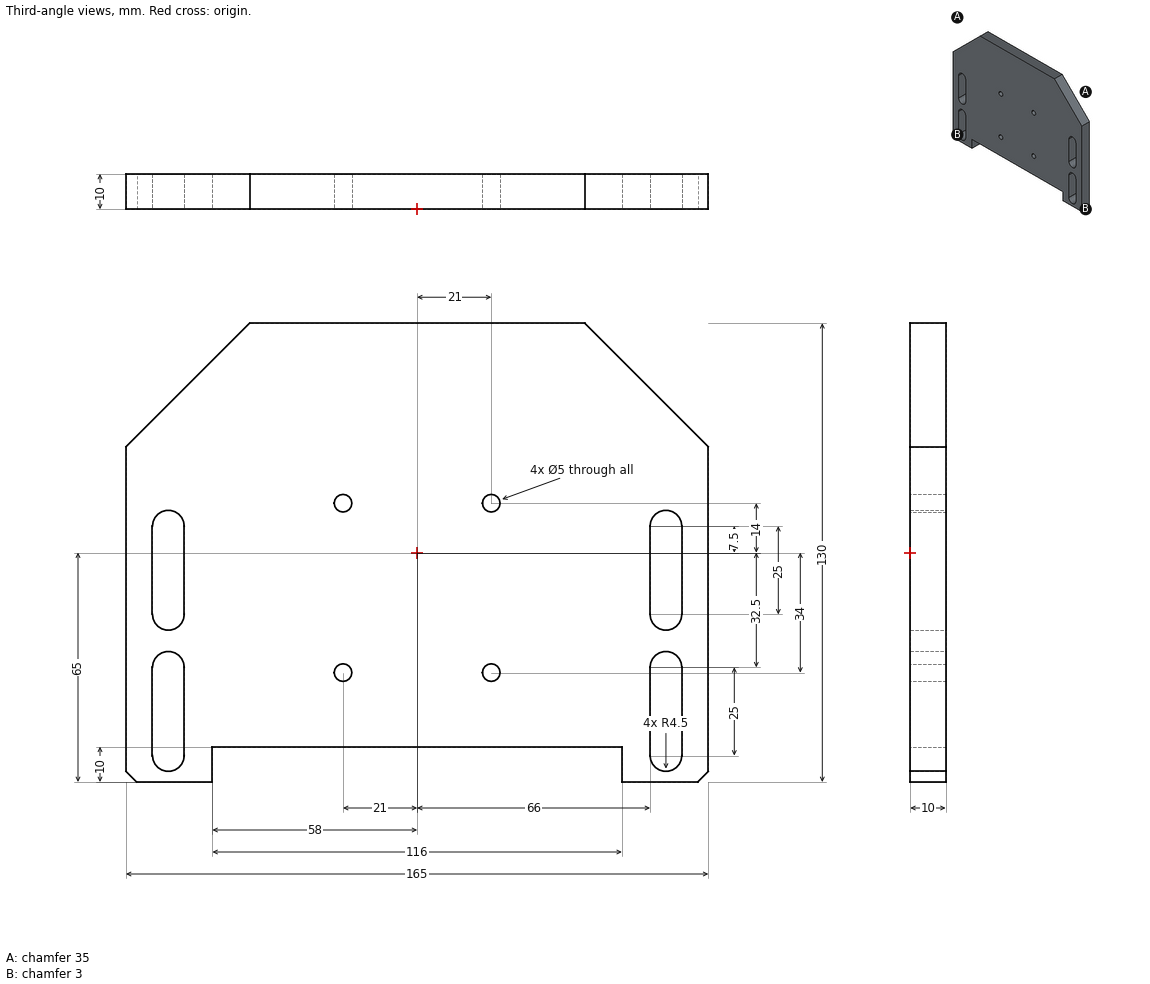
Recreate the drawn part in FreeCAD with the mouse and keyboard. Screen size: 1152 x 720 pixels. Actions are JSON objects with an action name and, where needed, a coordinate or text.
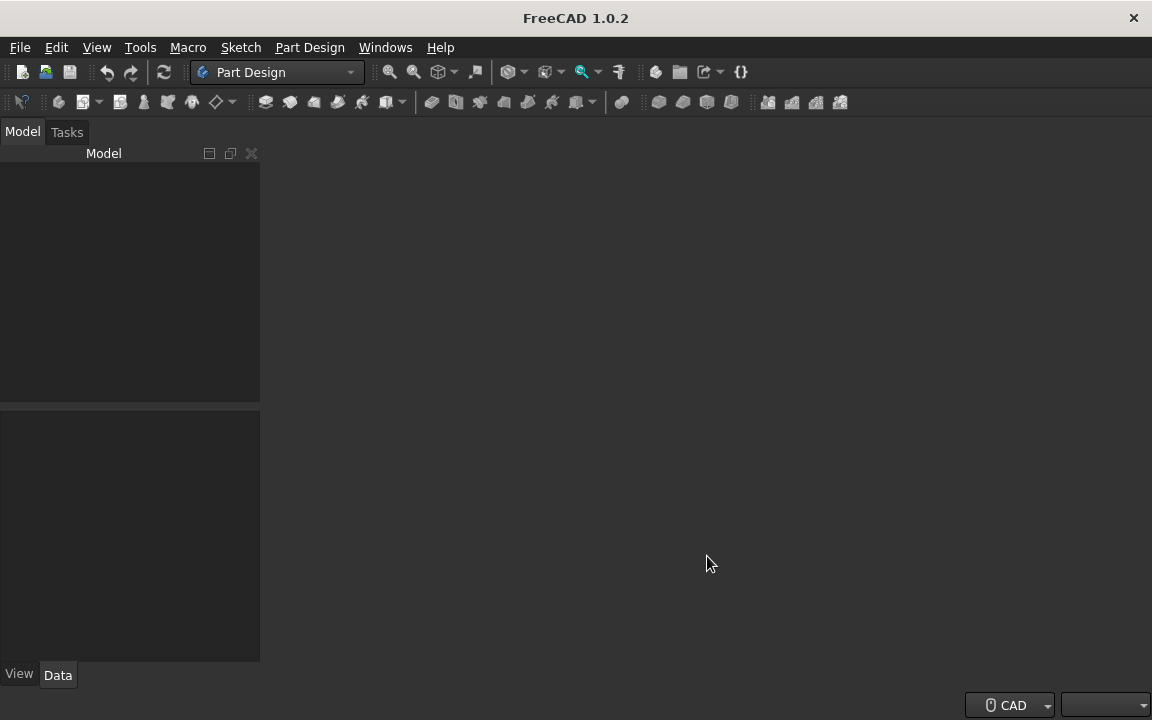
{"action": "key", "text": "ctrl+n"}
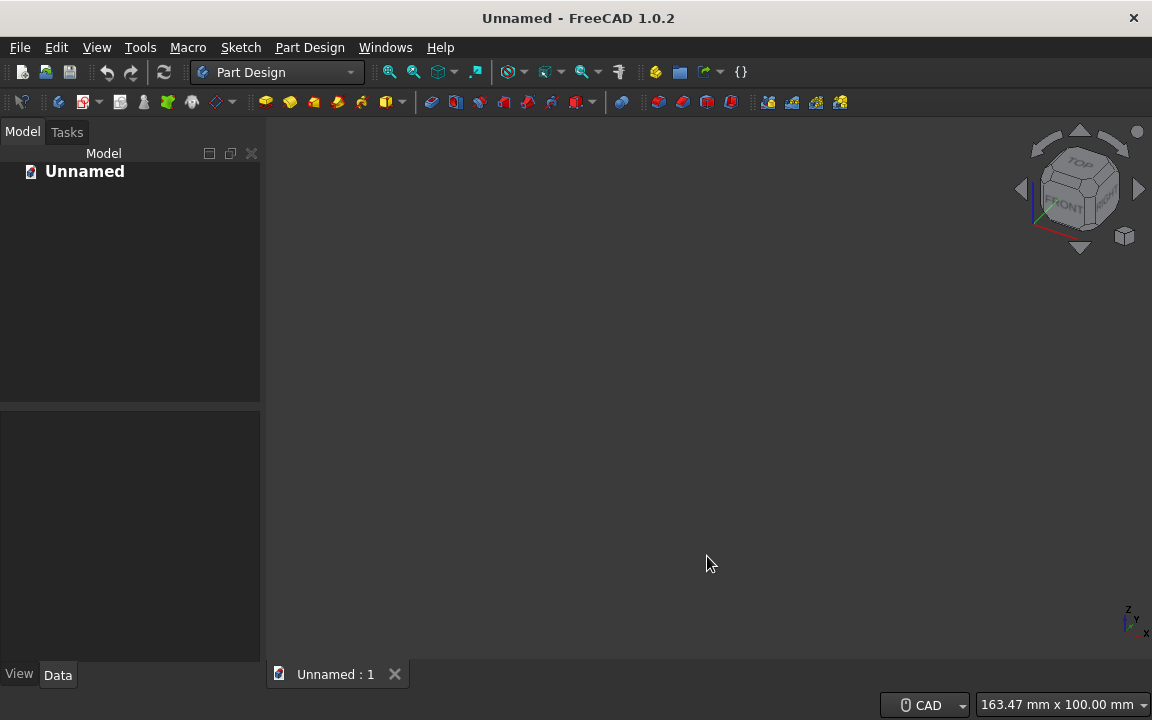
{"action": "left_click", "coordinate": [84, 102]}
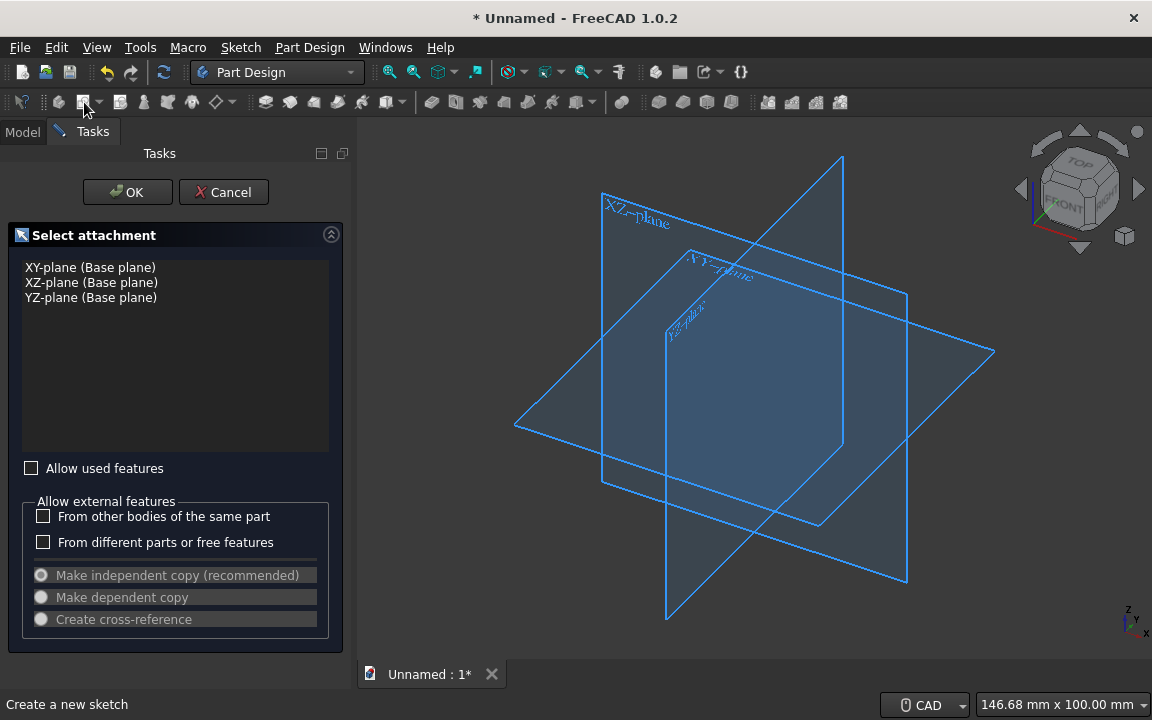
{"action": "left_click", "coordinate": [82, 282]}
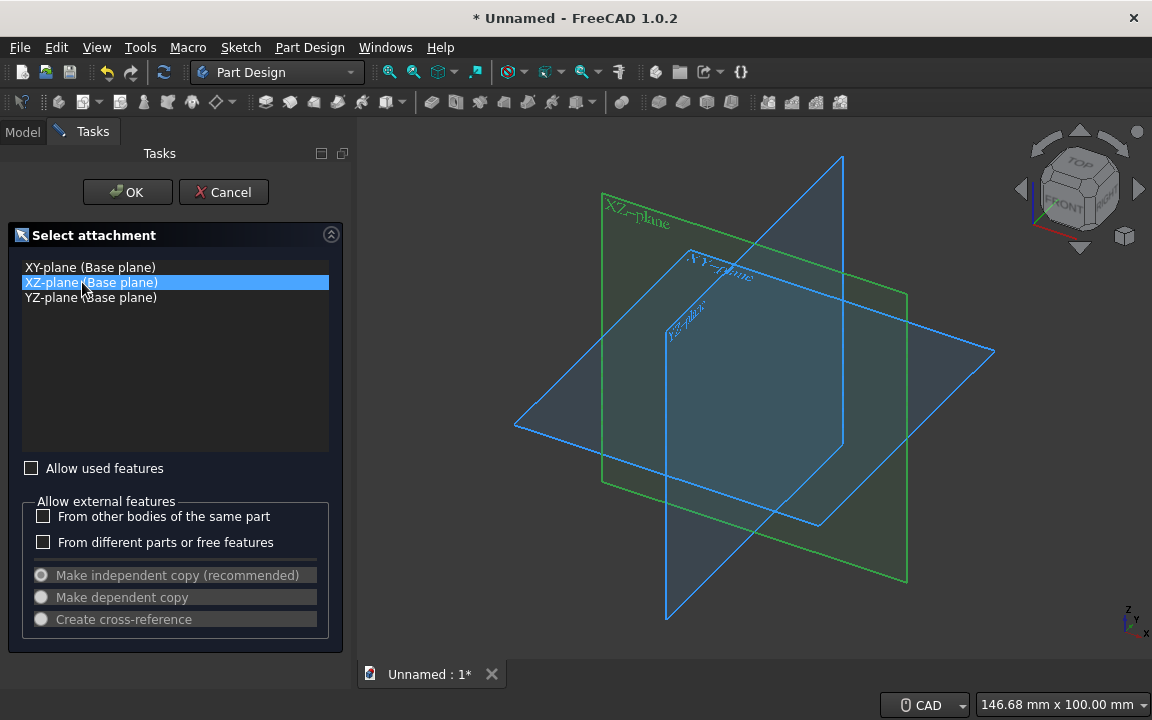
{"action": "left_click", "coordinate": [128, 192]}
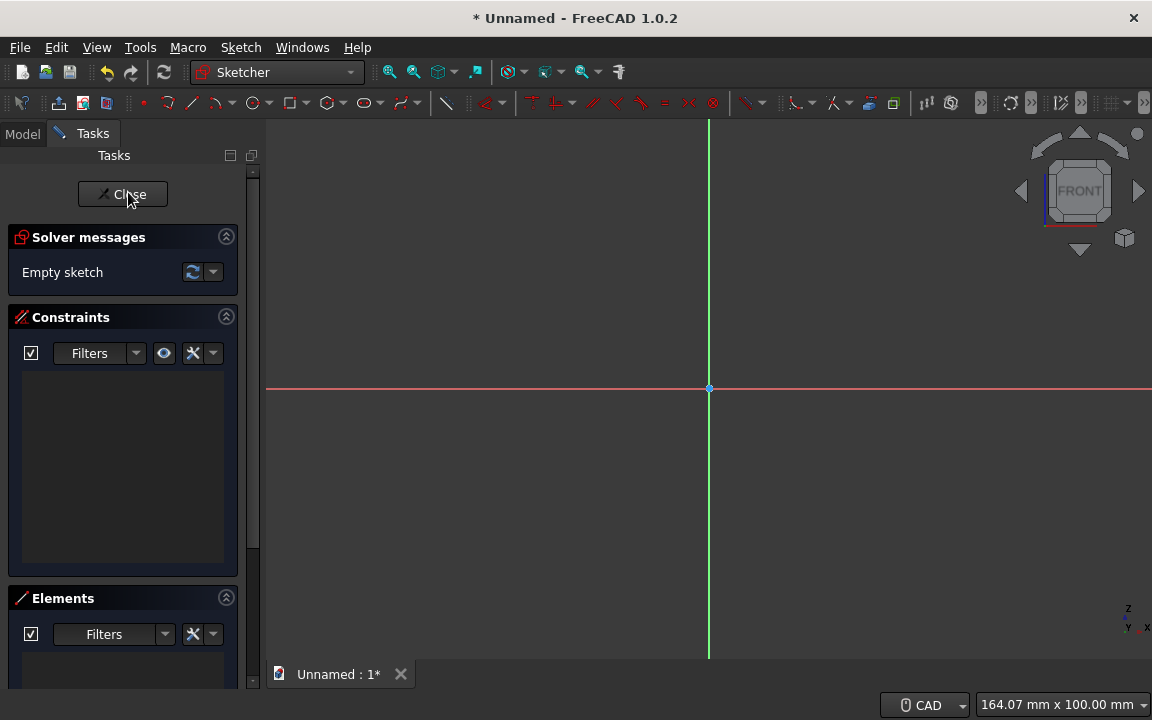
{"action": "scroll", "coordinate": [585, 389], "scroll_direction": "down", "scroll_amount": 4}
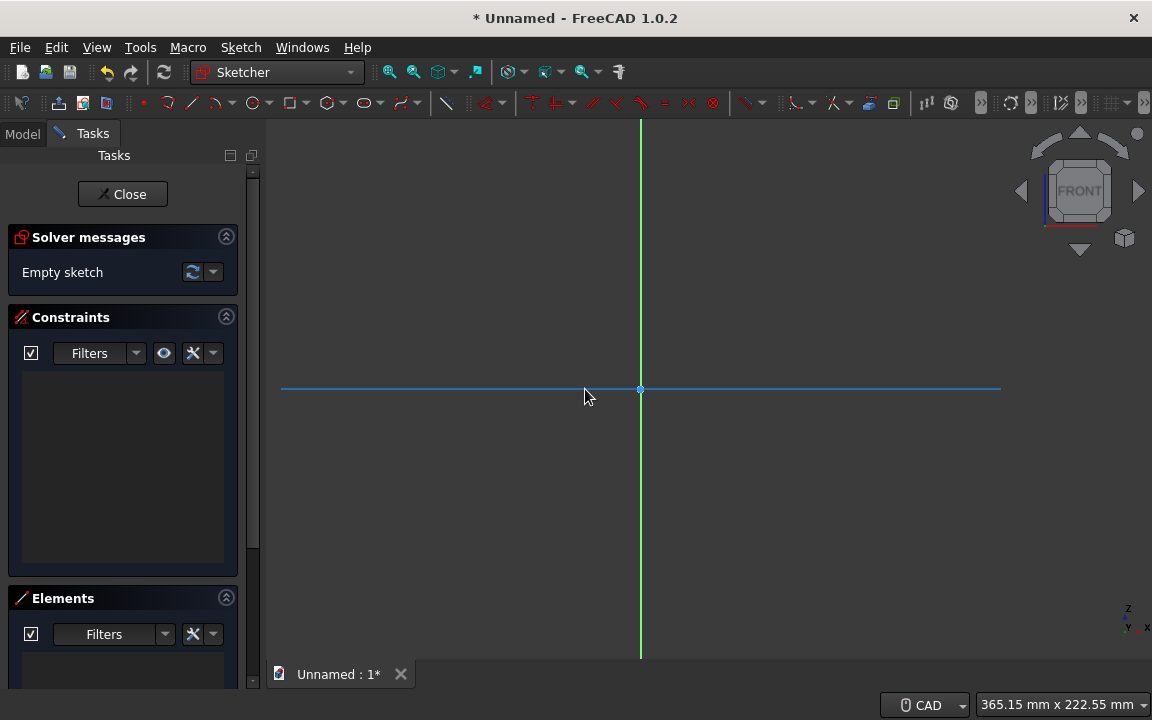
{"action": "left_click", "coordinate": [308, 104]}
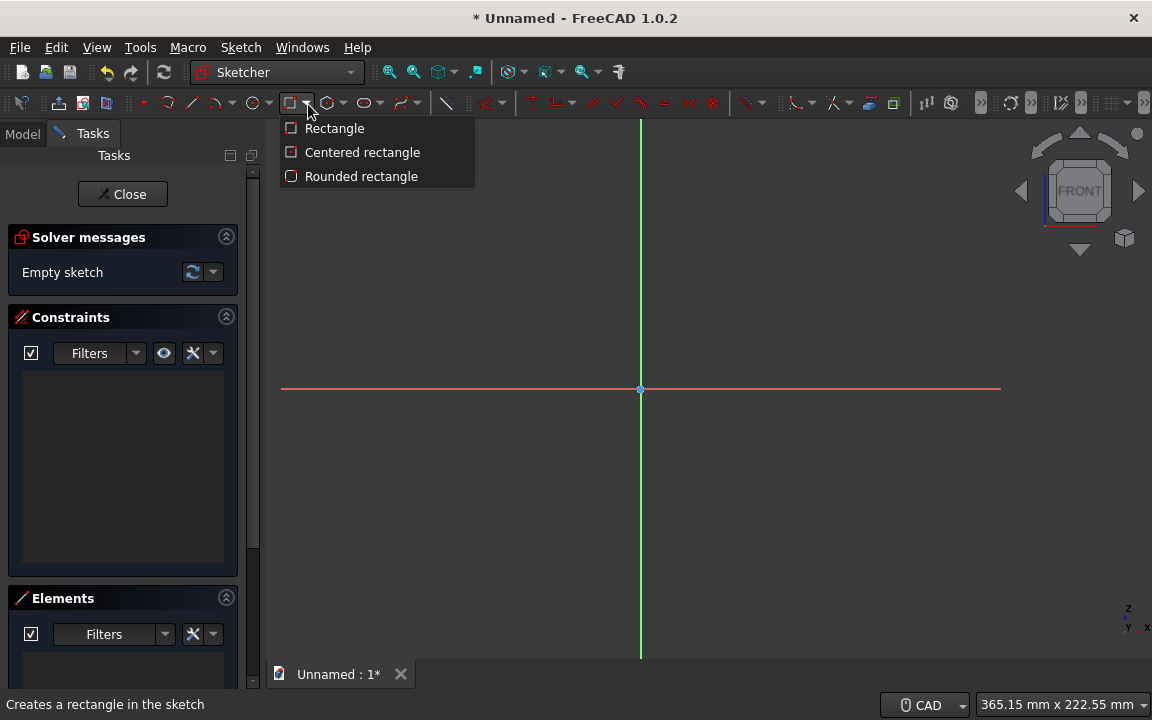
{"action": "left_click", "coordinate": [378, 152]}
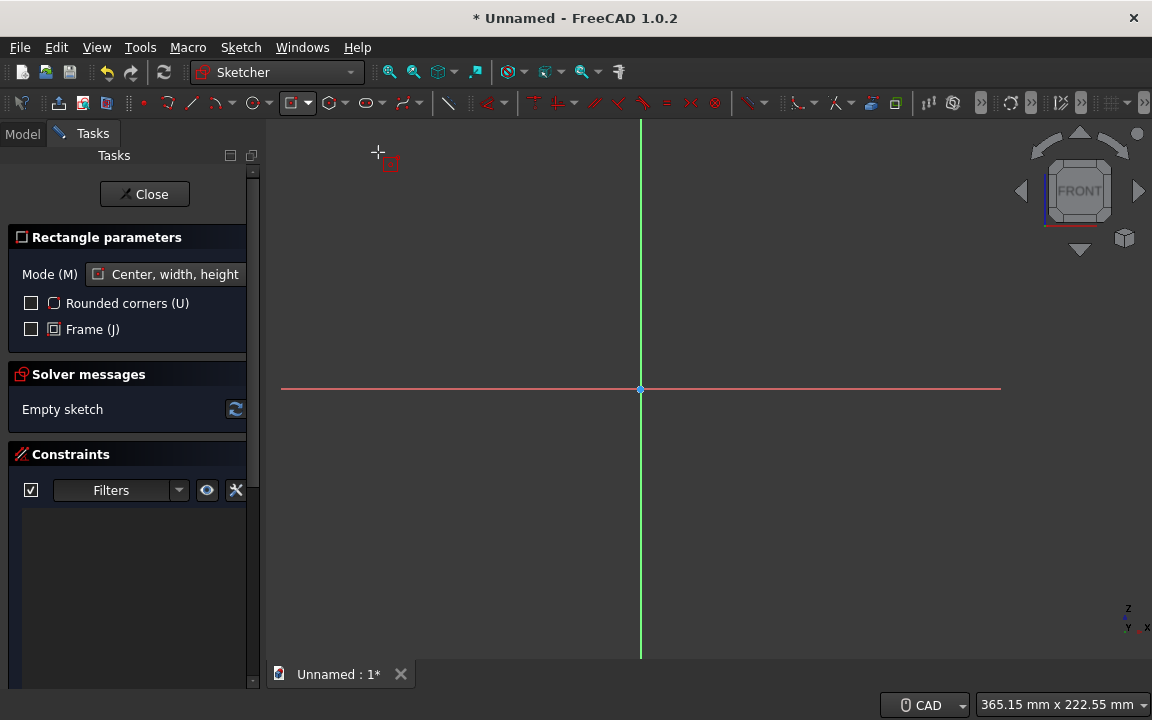
{"action": "left_click", "coordinate": [641, 389]}
{"action": "left_click", "coordinate": [841, 232]}
{"action": "key", "text": "Escape"}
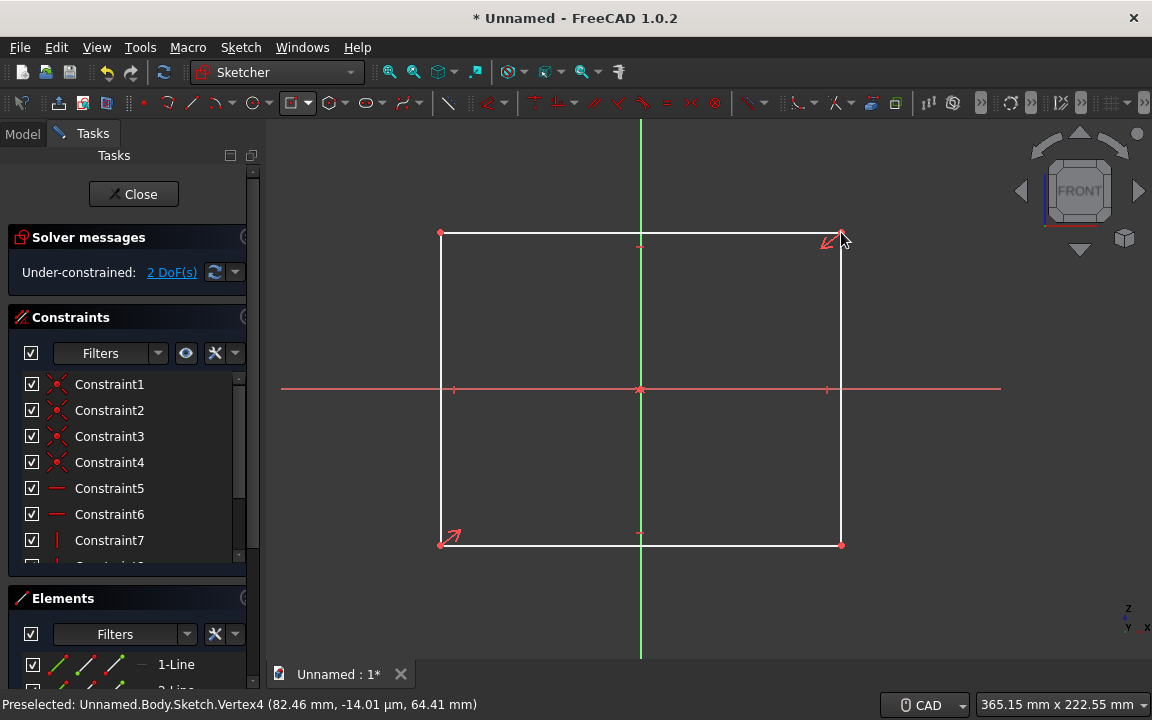
{"action": "key", "text": "d"}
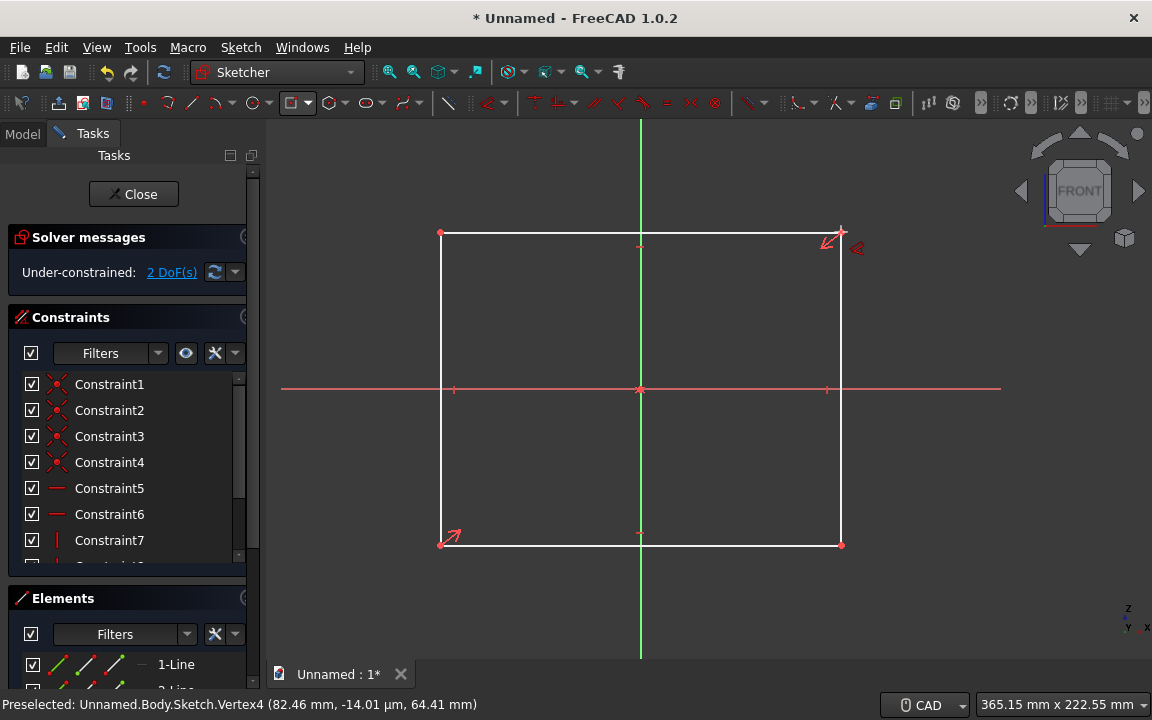
{"action": "left_click", "coordinate": [561, 546]}
{"action": "left_click", "coordinate": [549, 580]}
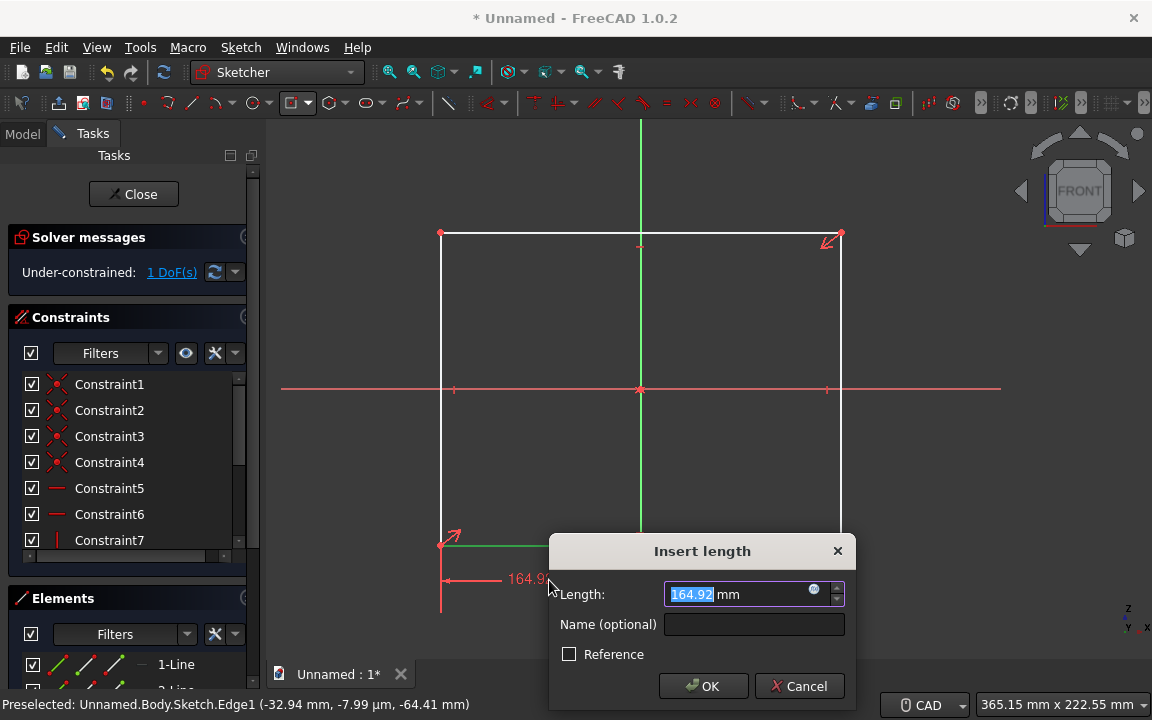
{"action": "type", "text": "165"}
{"action": "key", "text": "Return"}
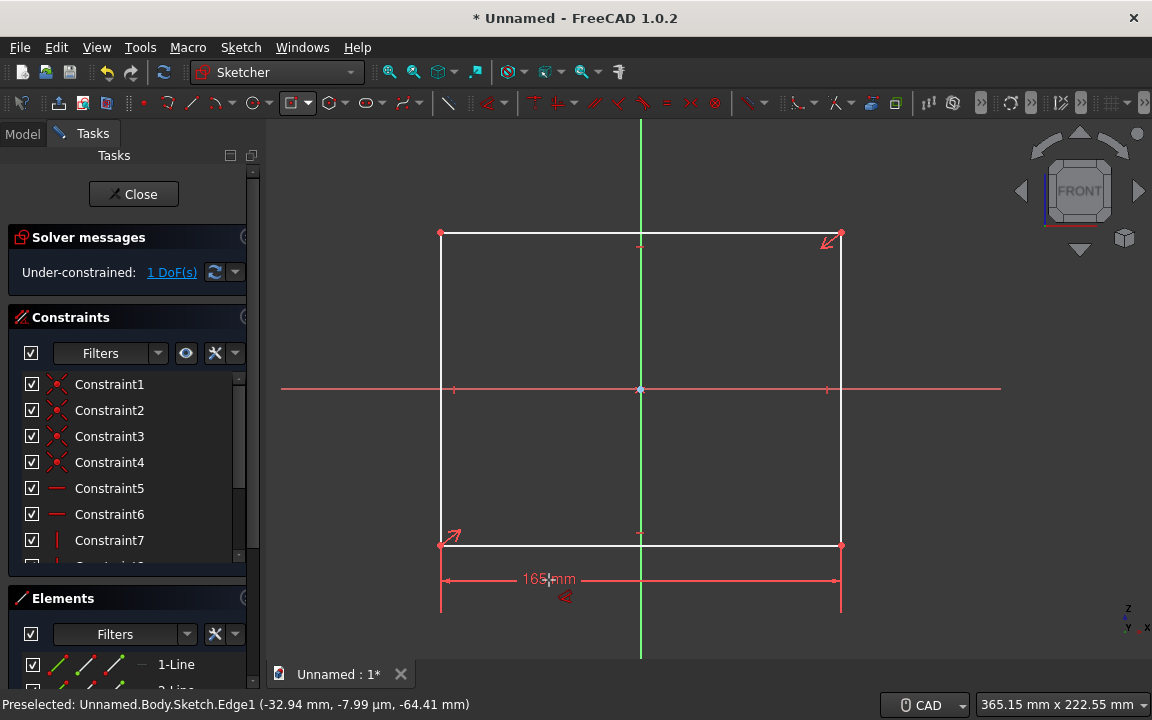
{"action": "left_click", "coordinate": [841, 452]}
{"action": "left_click", "coordinate": [875, 317]}